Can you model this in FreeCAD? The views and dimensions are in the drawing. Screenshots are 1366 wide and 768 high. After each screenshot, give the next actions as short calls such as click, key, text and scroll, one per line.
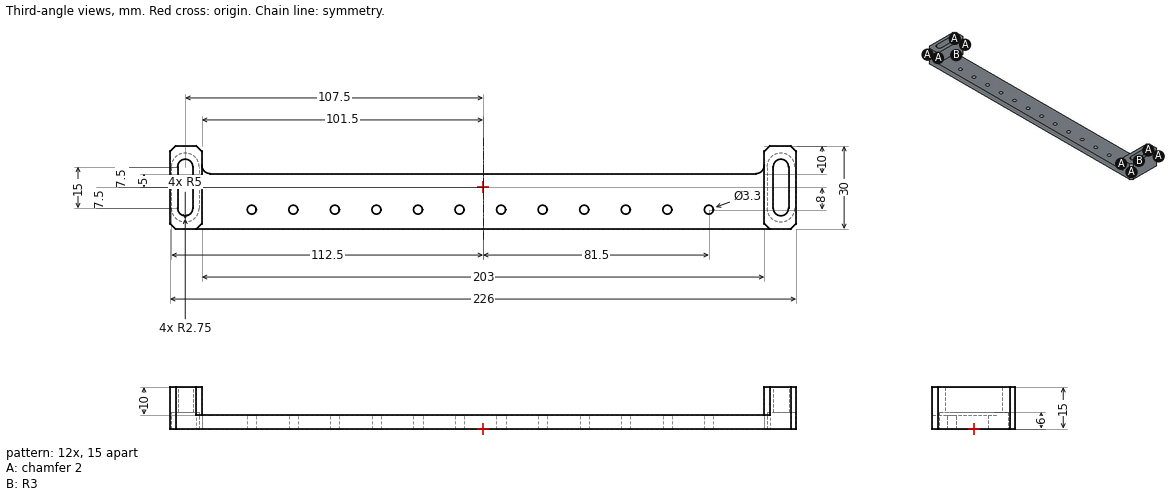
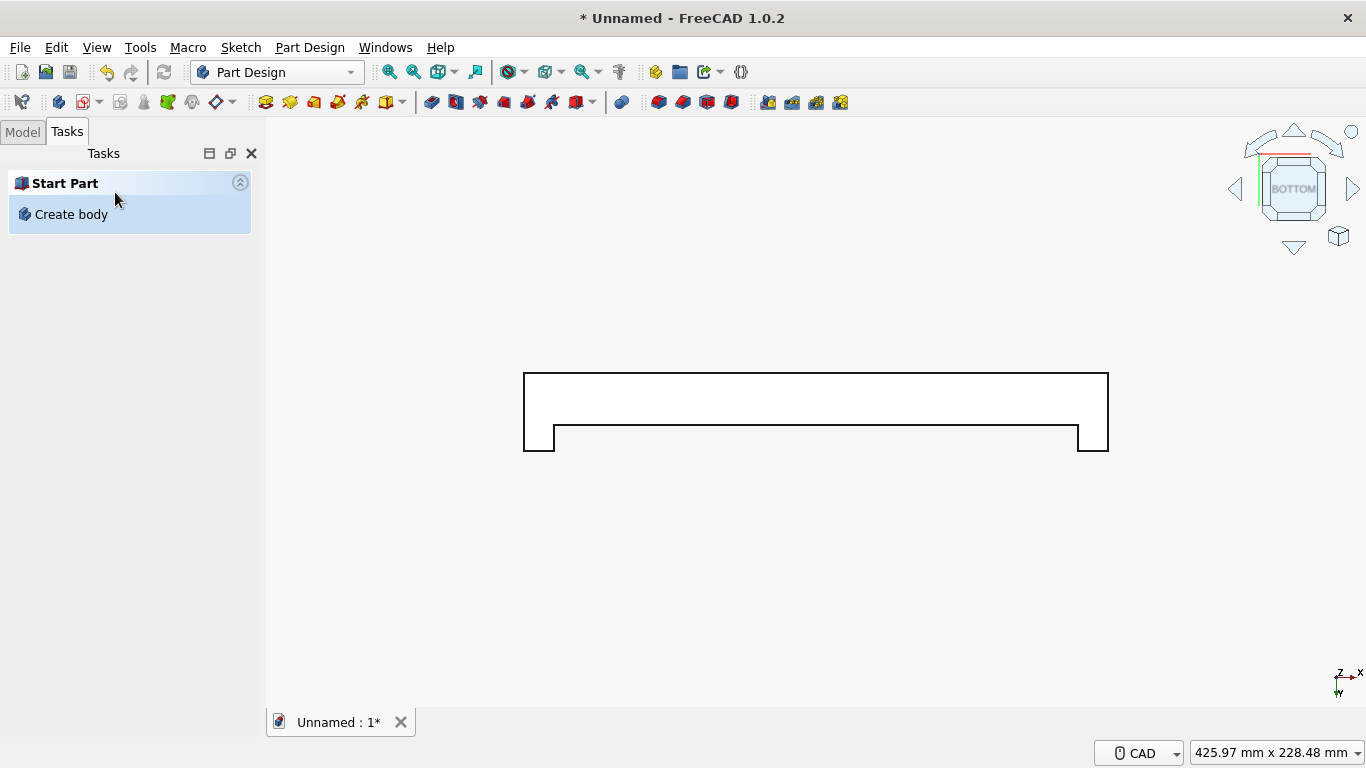
click(1066, 400)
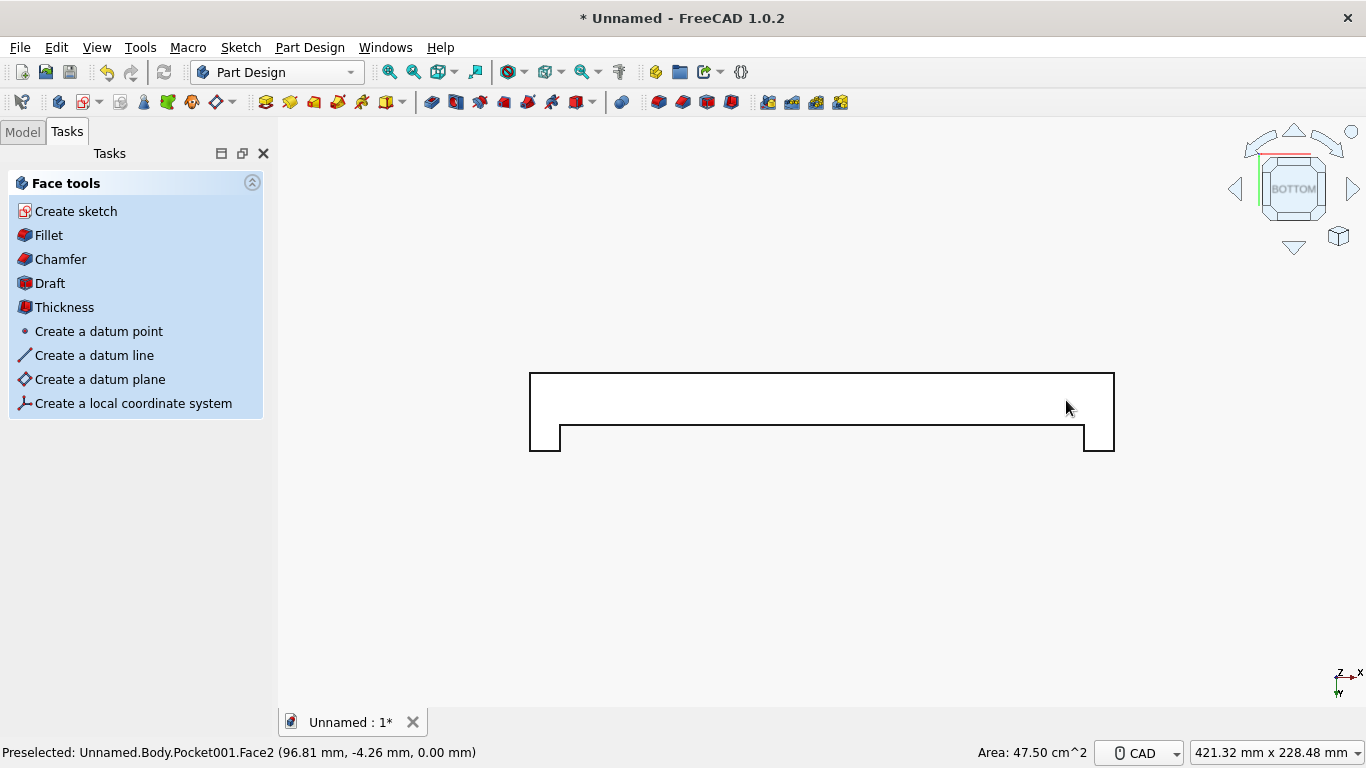
click(84, 102)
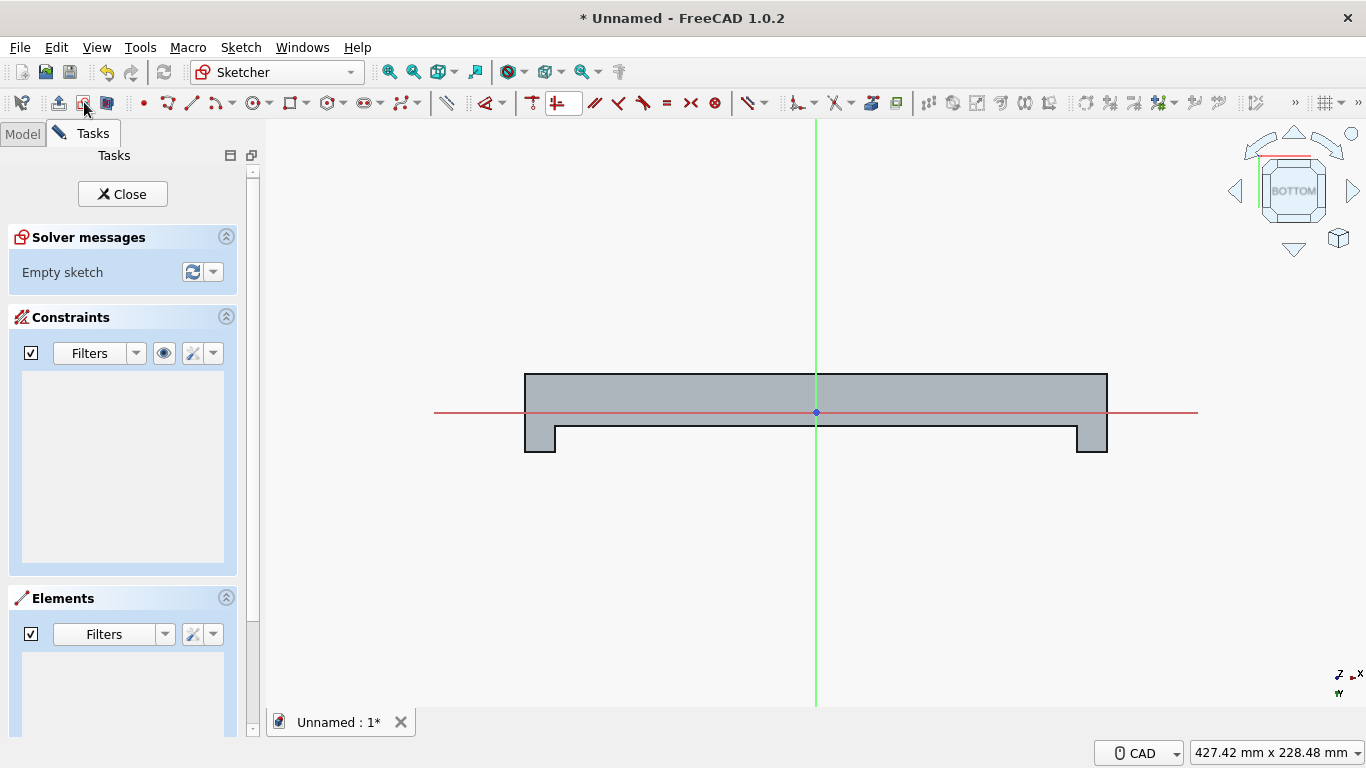
key(g)
key(s)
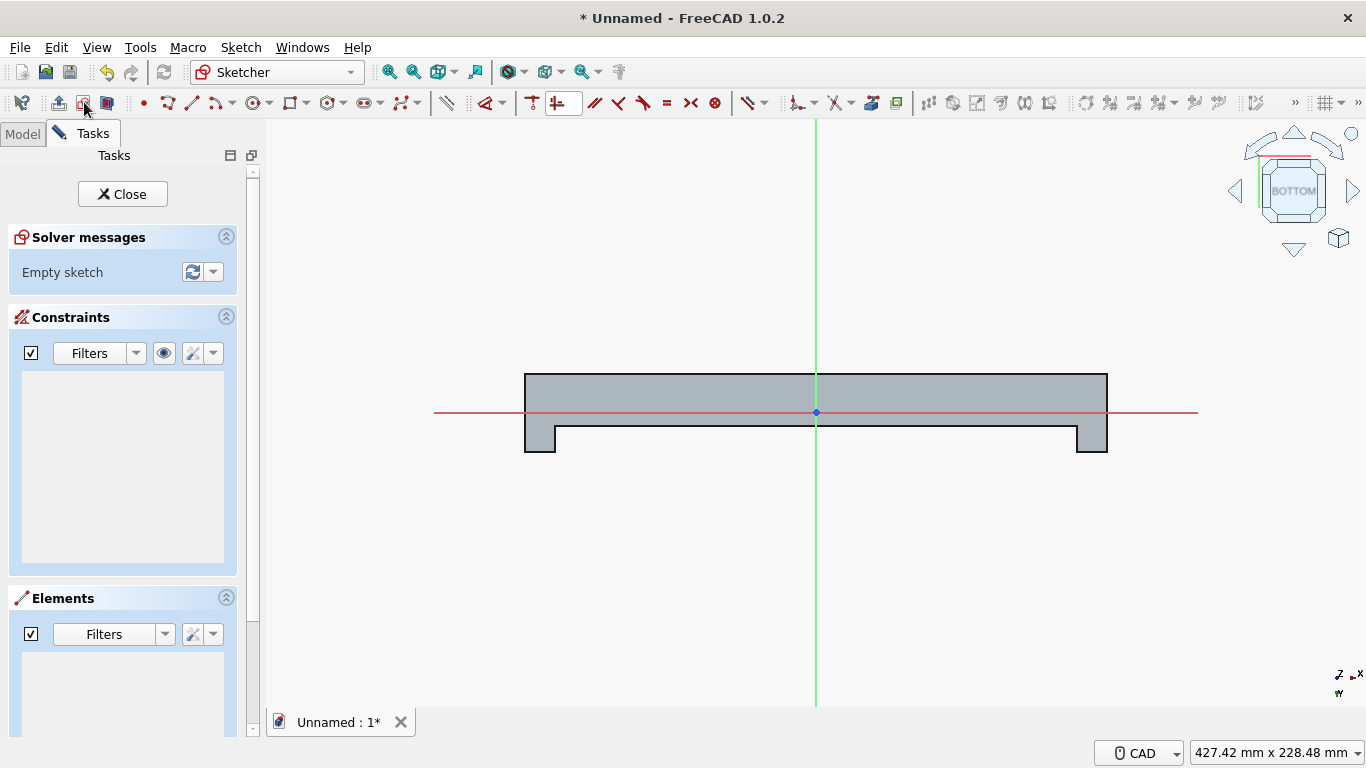
scroll(539, 432, up, 6)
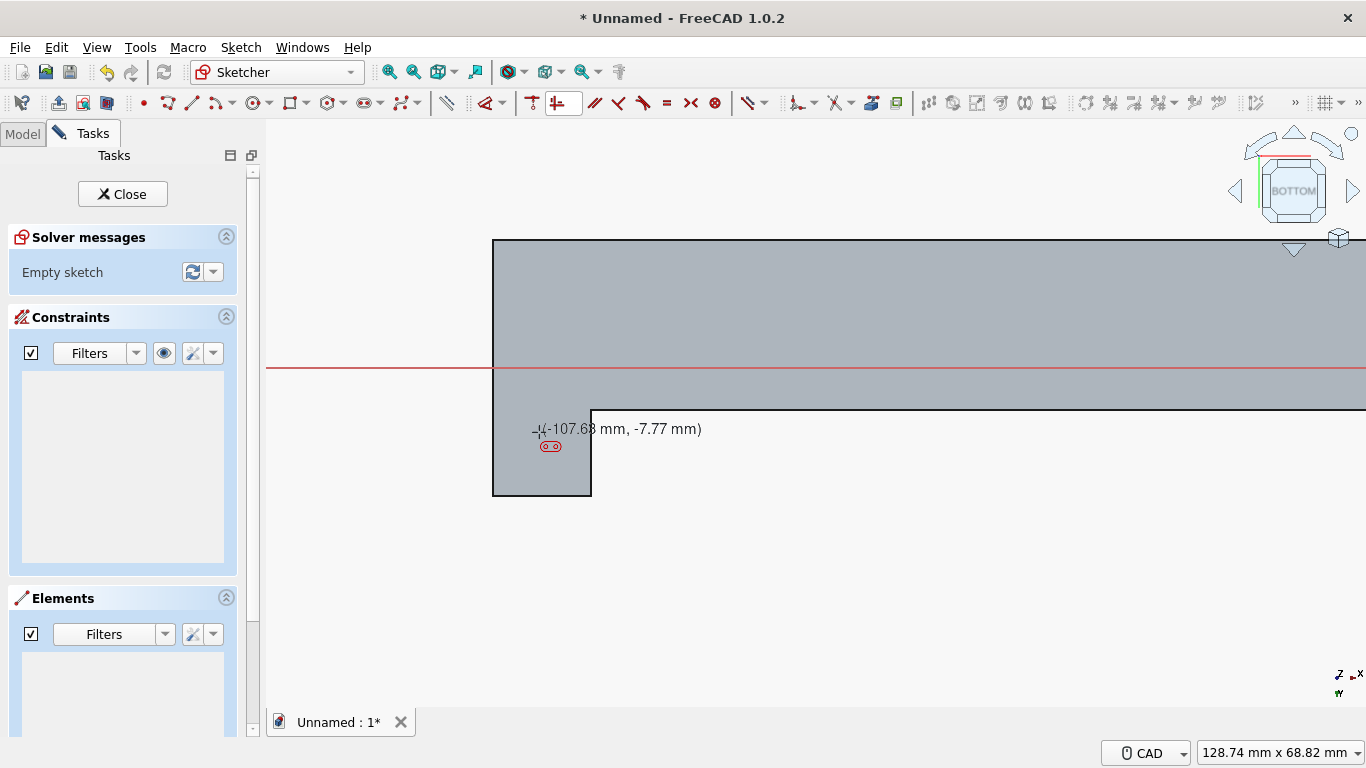
click(540, 432)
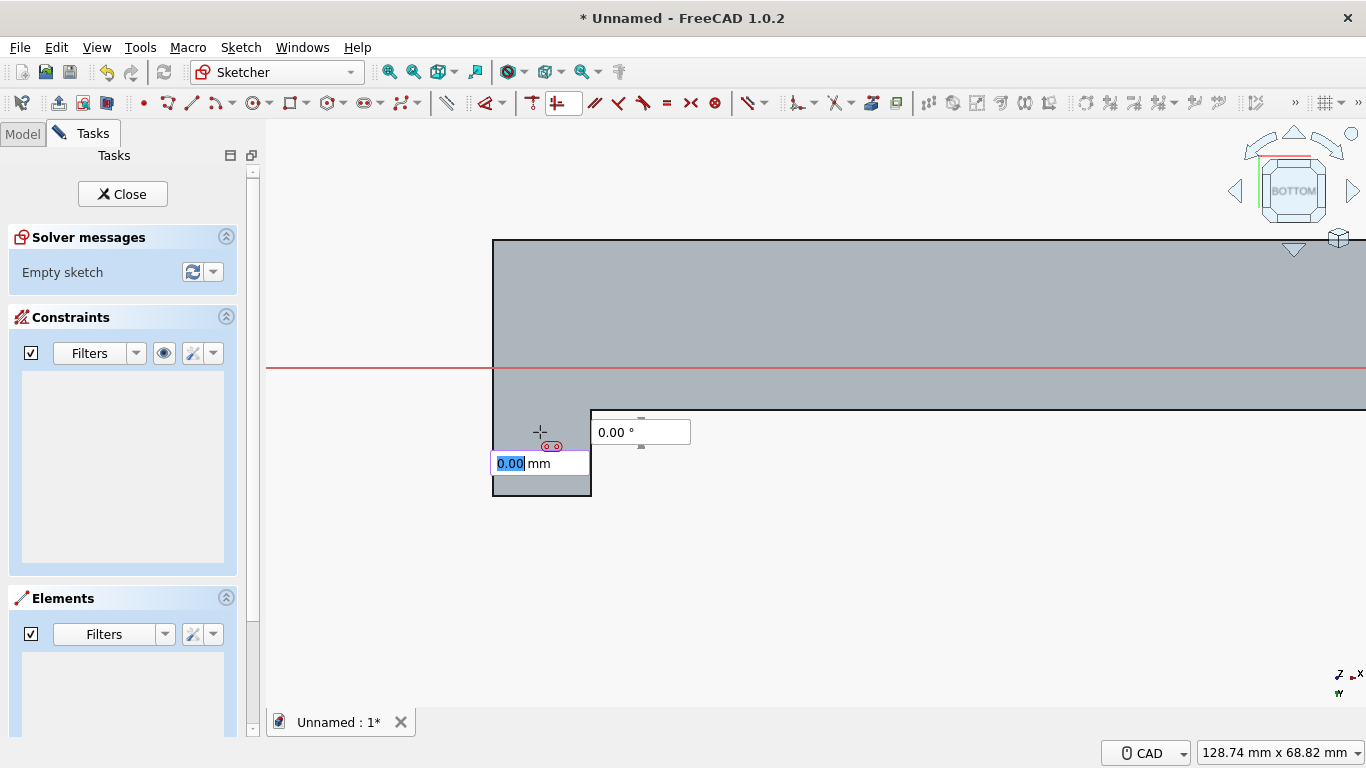
click(540, 304)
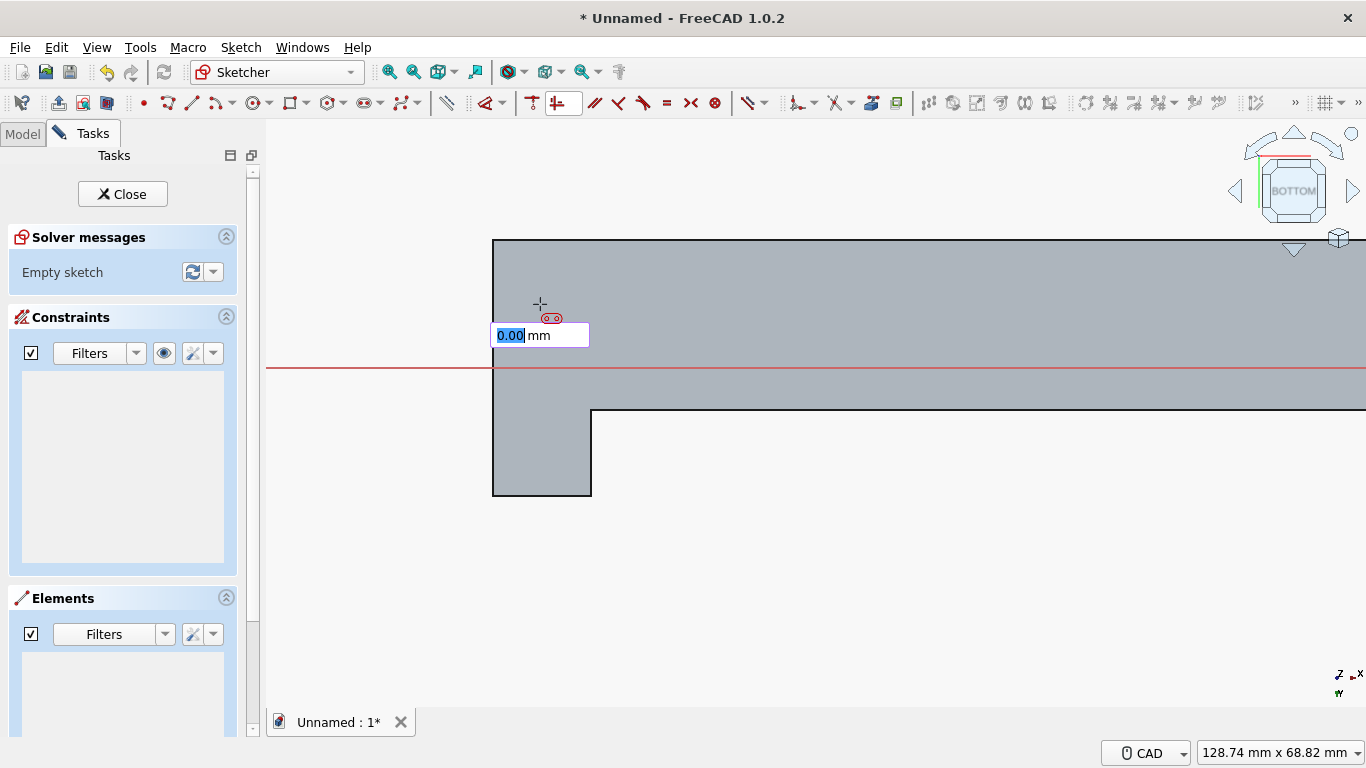
click(563, 387)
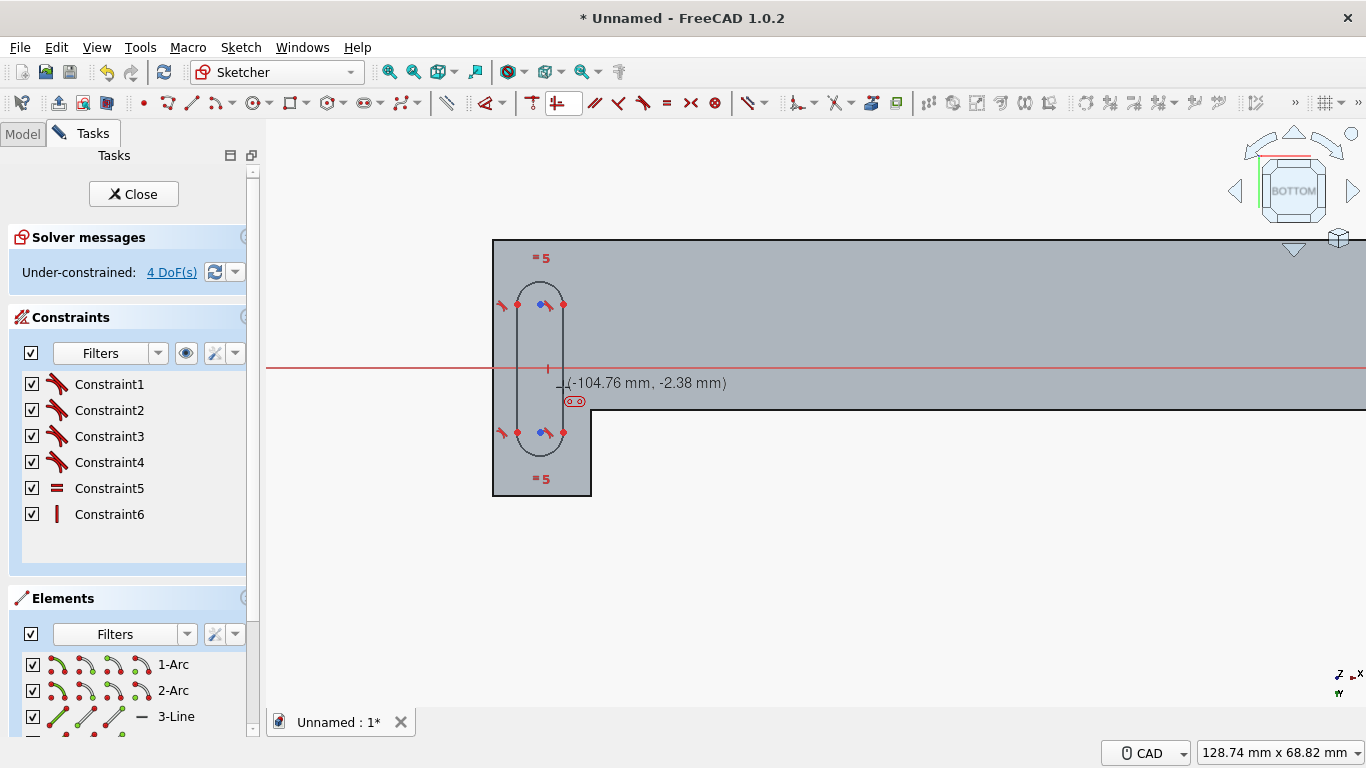
scroll(334, 439, down, 5)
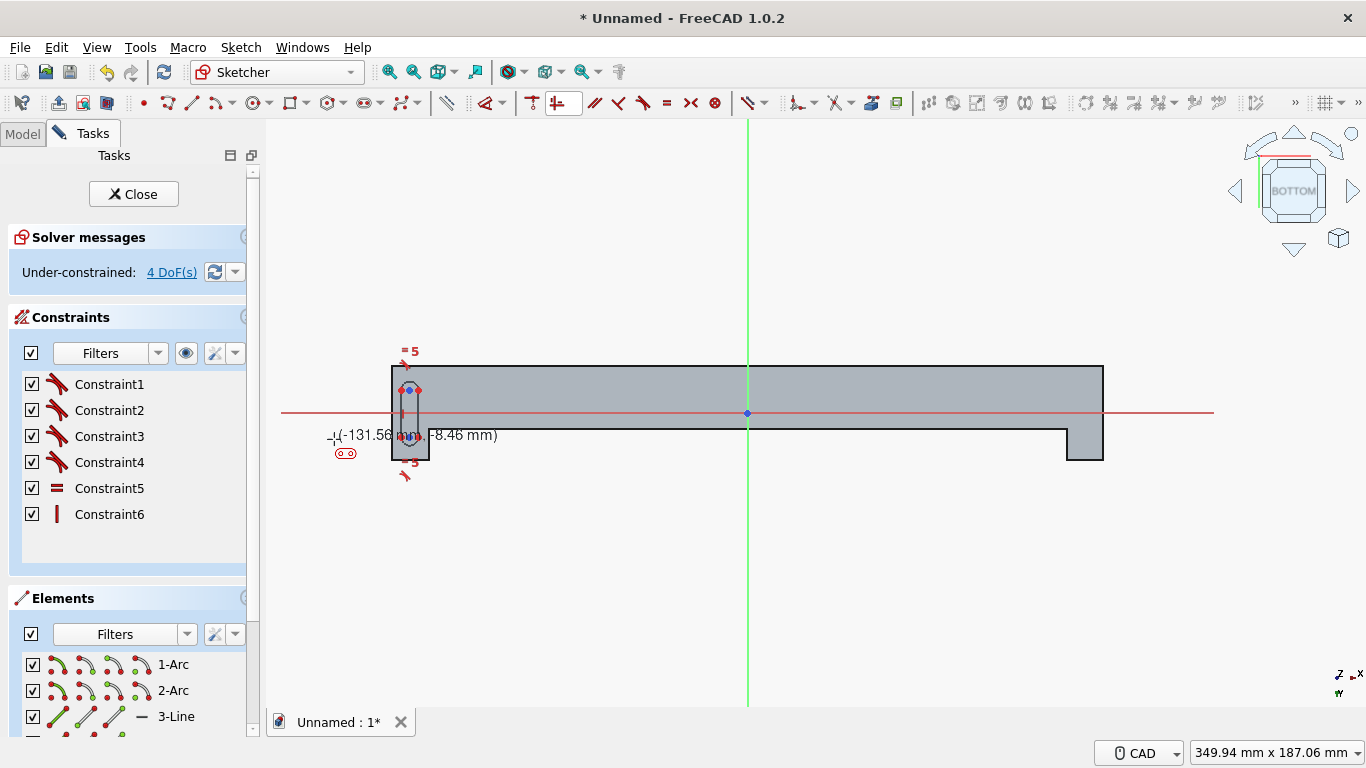
scroll(1085, 437, up, 5)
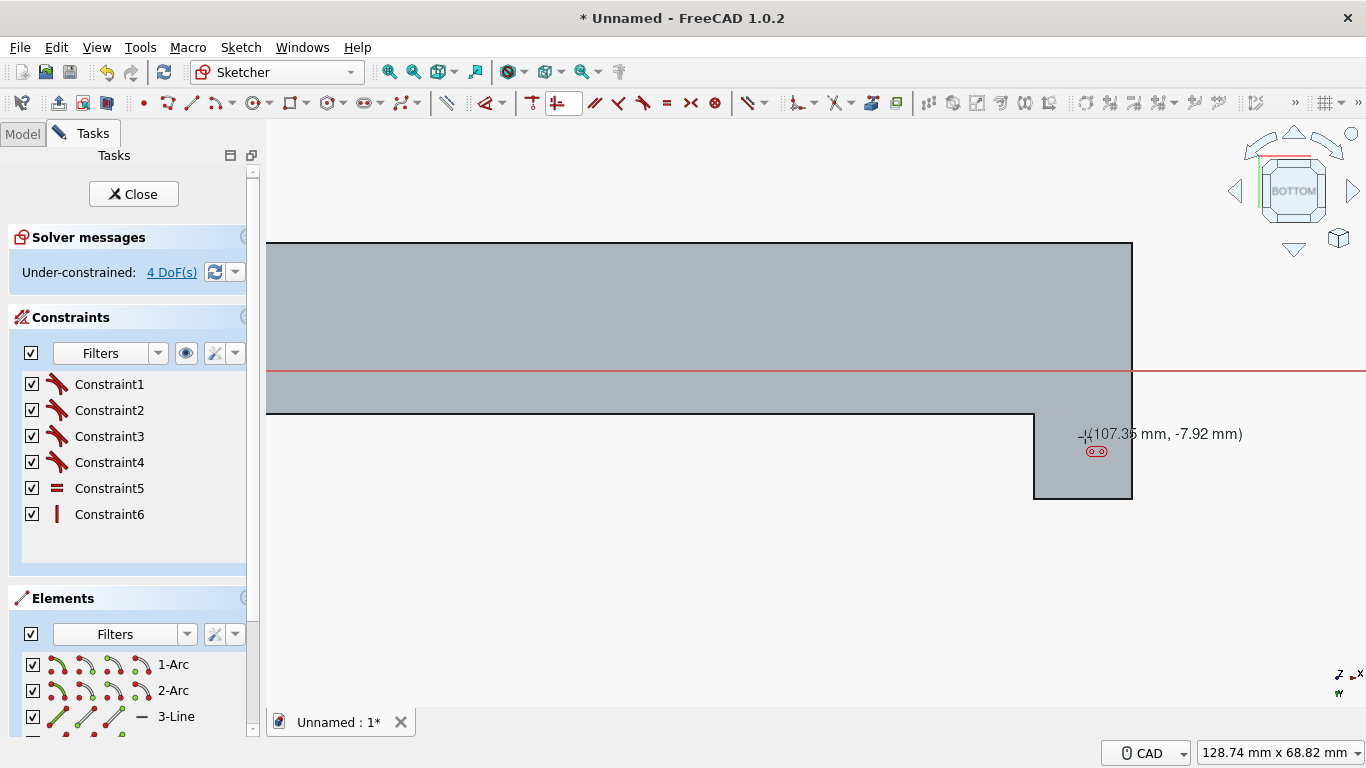
click(1085, 435)